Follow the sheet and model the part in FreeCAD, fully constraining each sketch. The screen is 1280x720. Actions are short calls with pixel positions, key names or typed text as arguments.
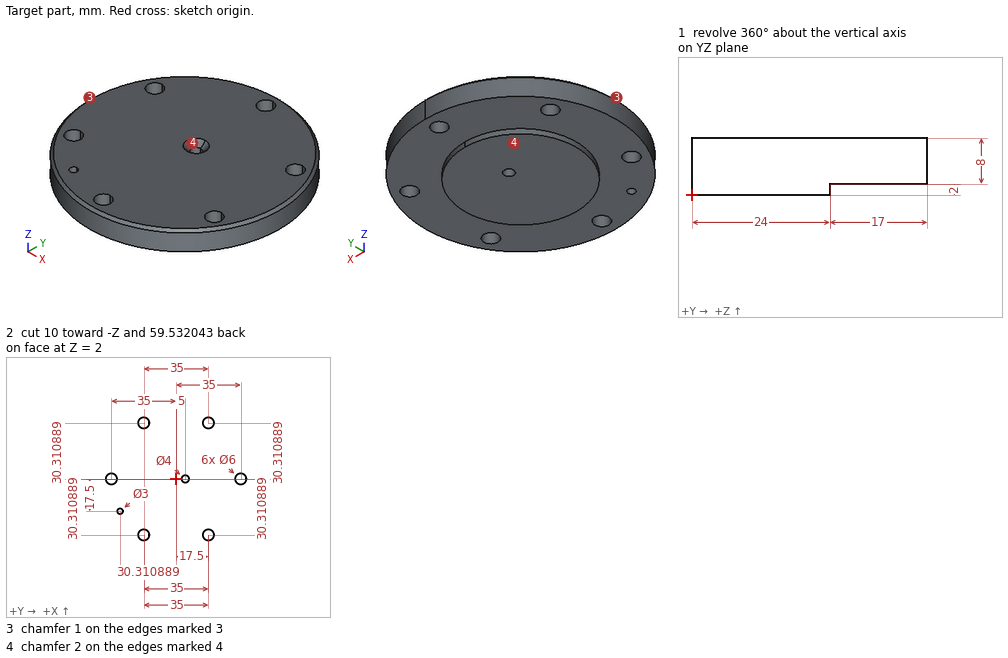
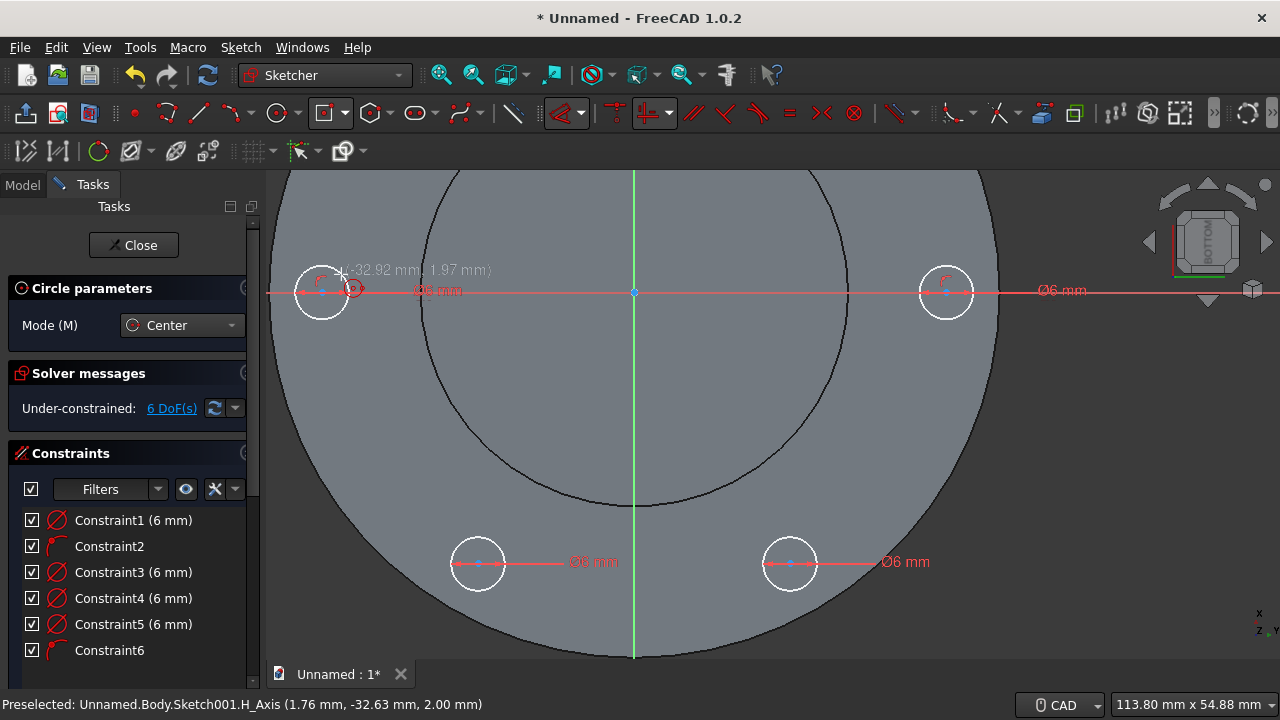
scroll(790, 563, down, 3)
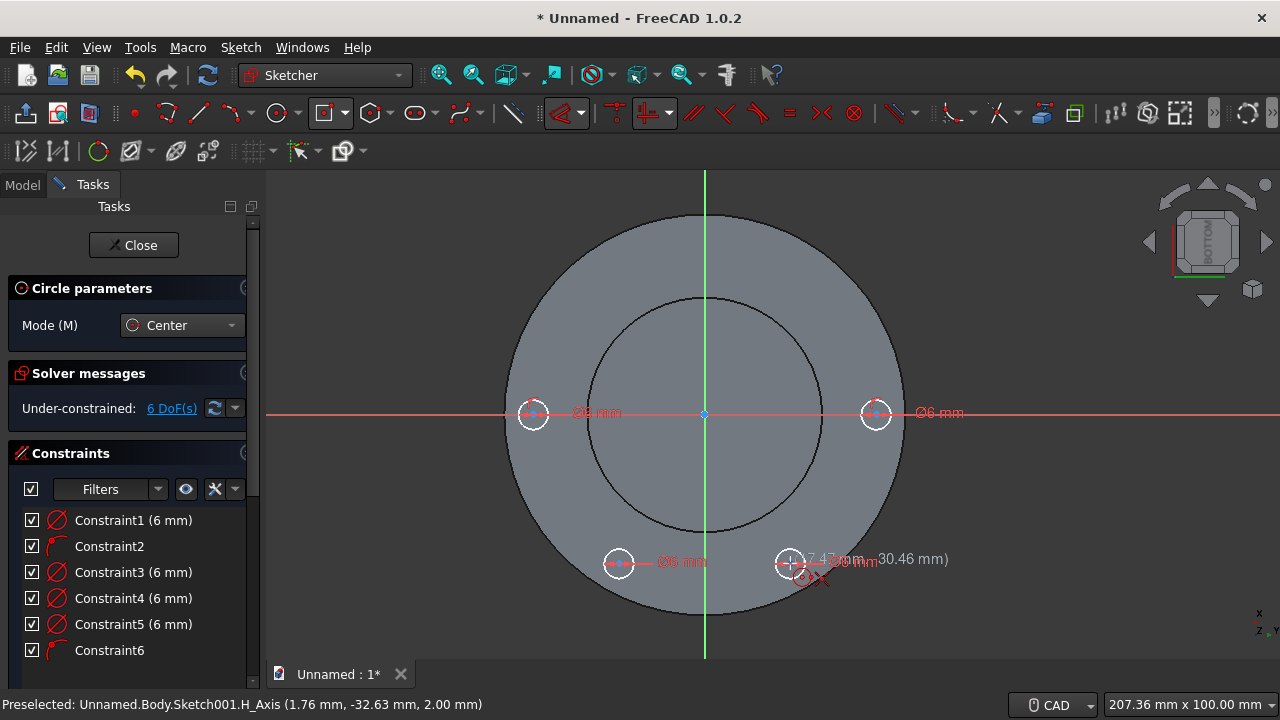
scroll(619, 267, up, 3)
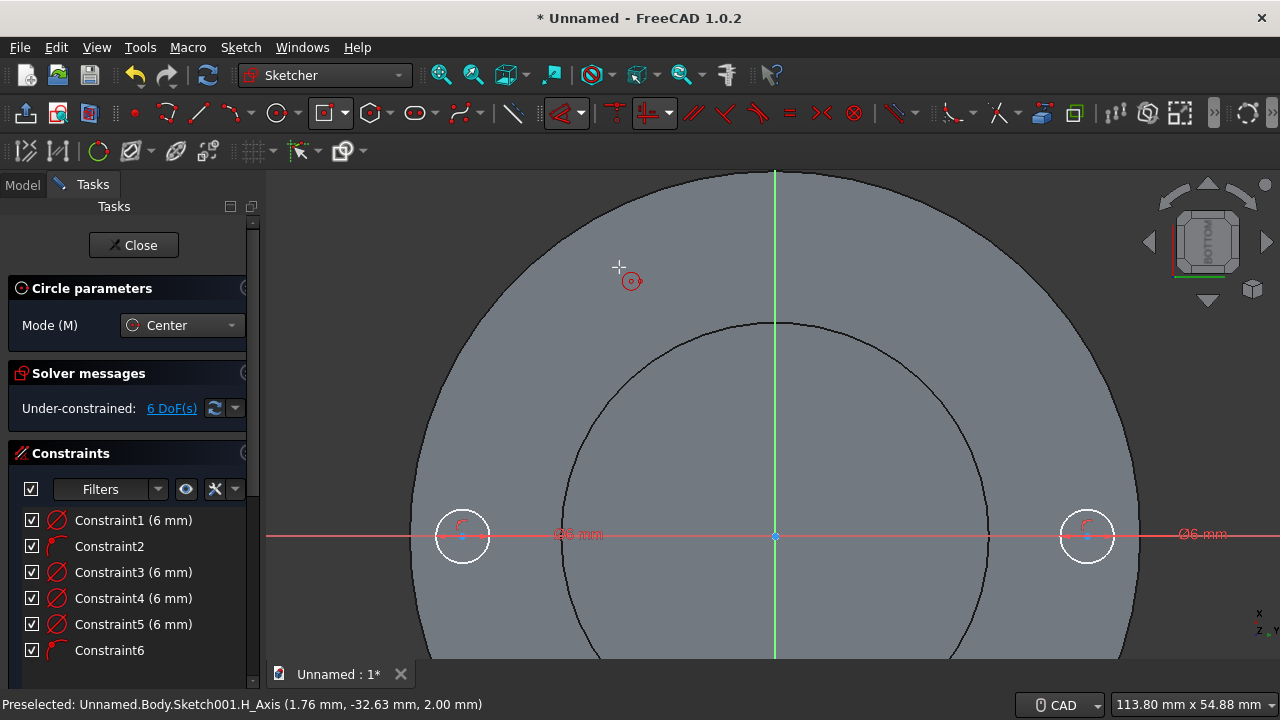
click(619, 266)
move(638, 247)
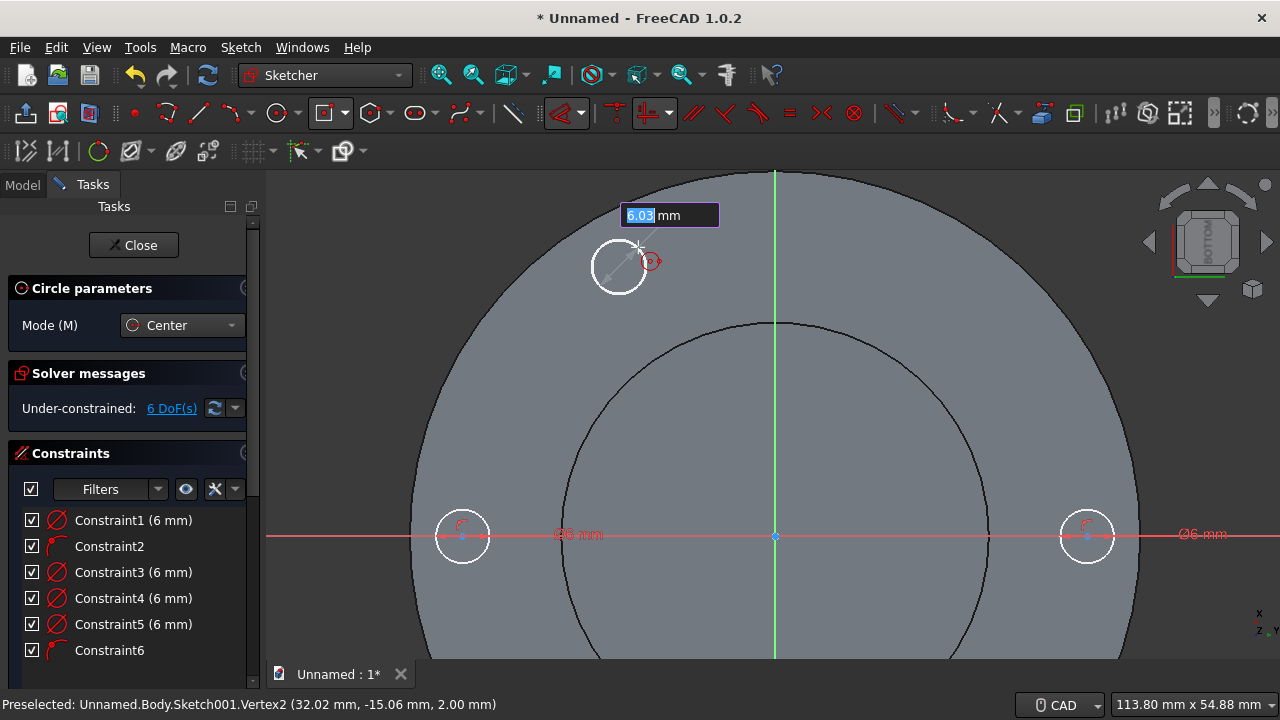
text(6)
key(Return)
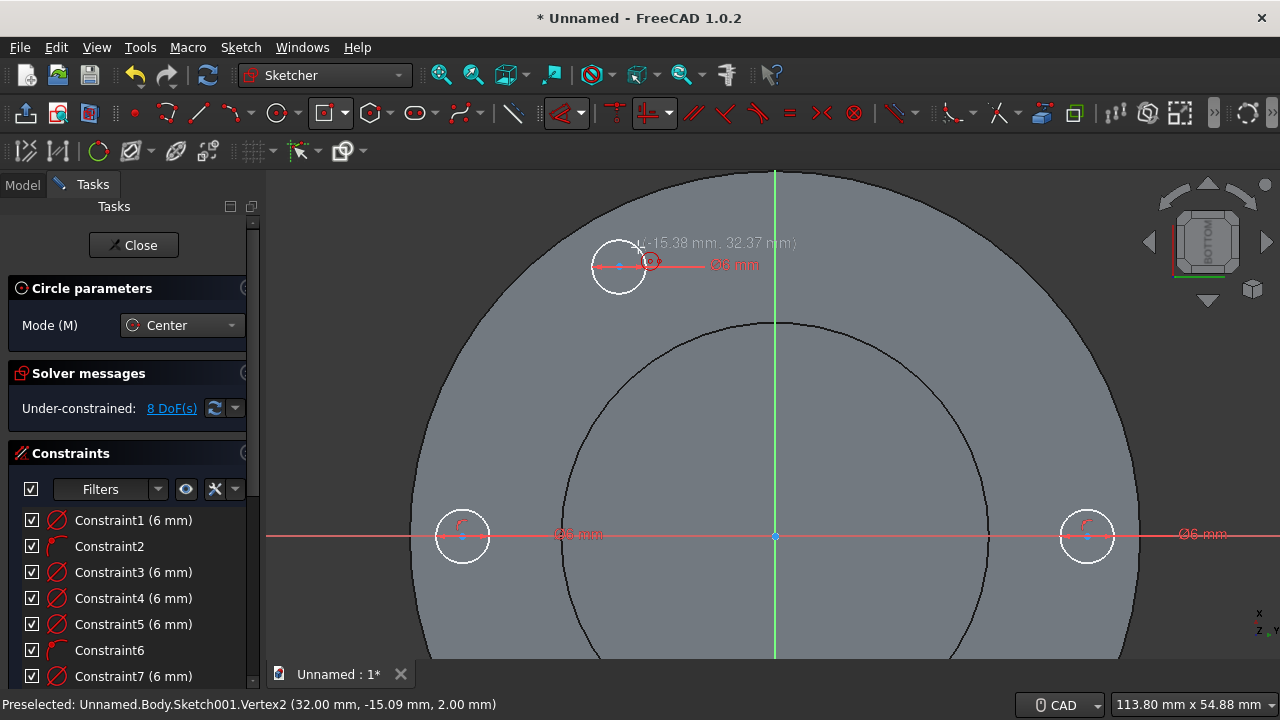
click(931, 266)
move(950, 247)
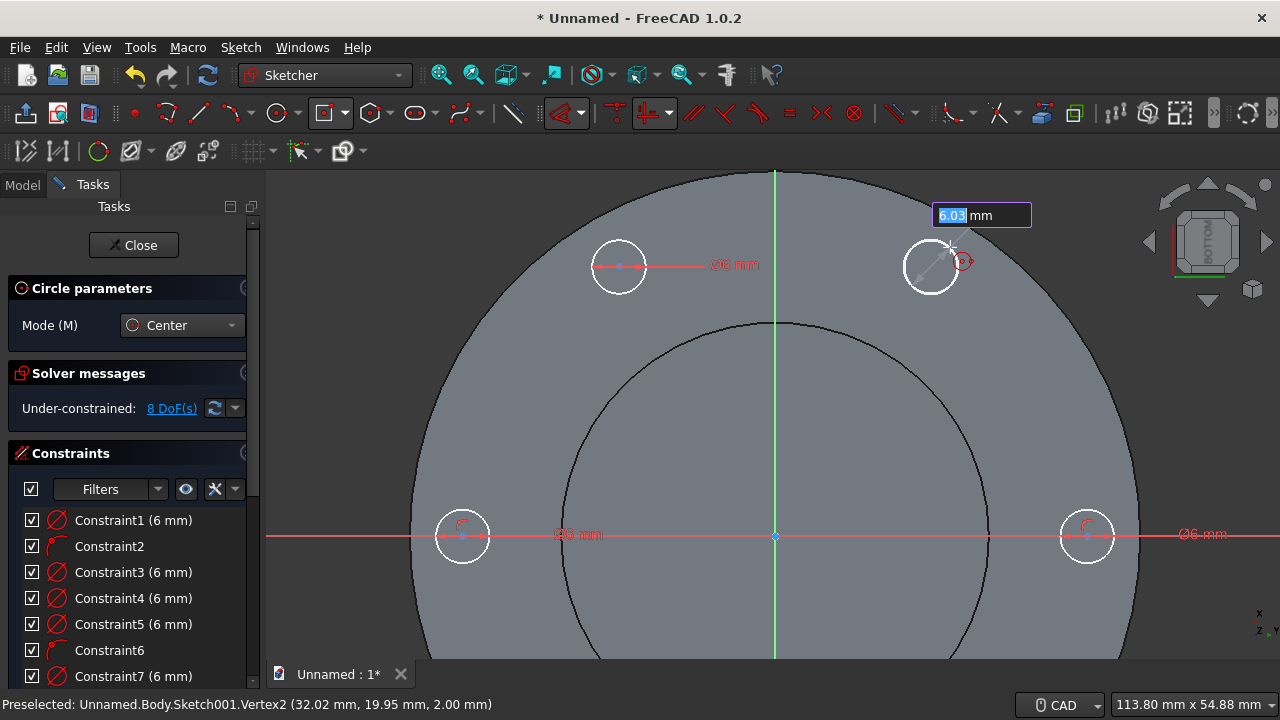
text(6)
key(Return)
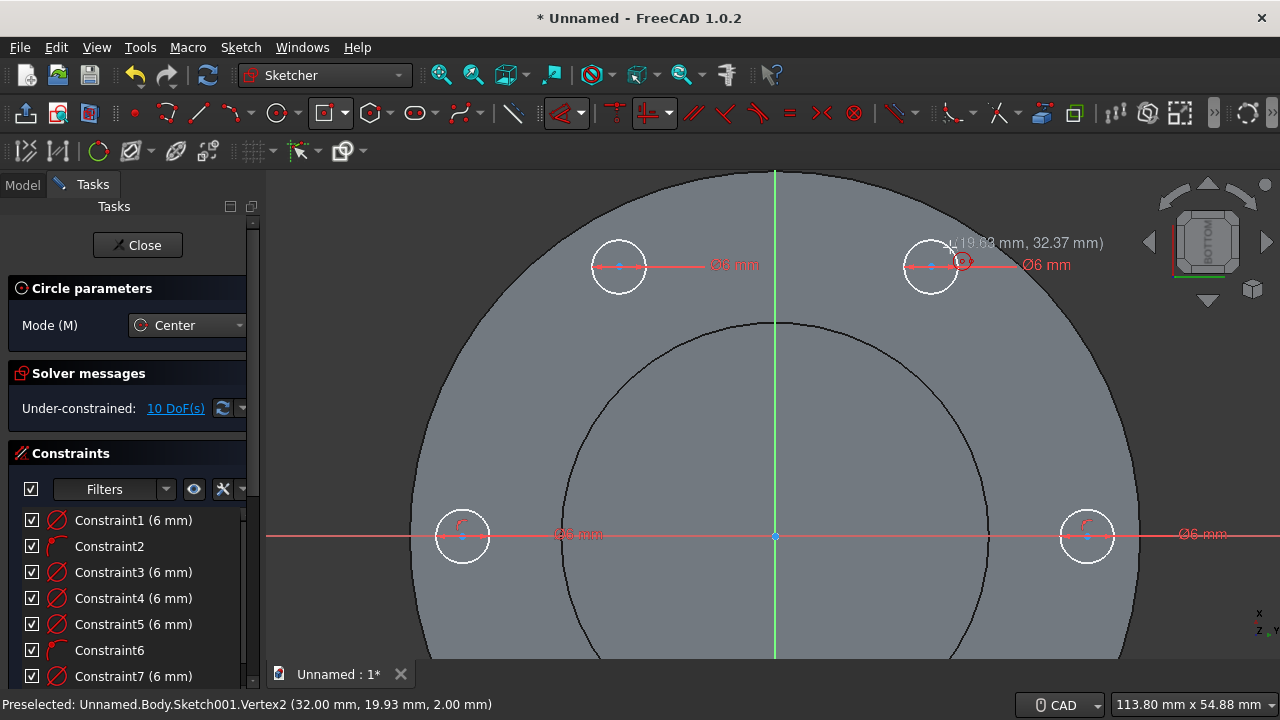
scroll(619, 266, down, 3)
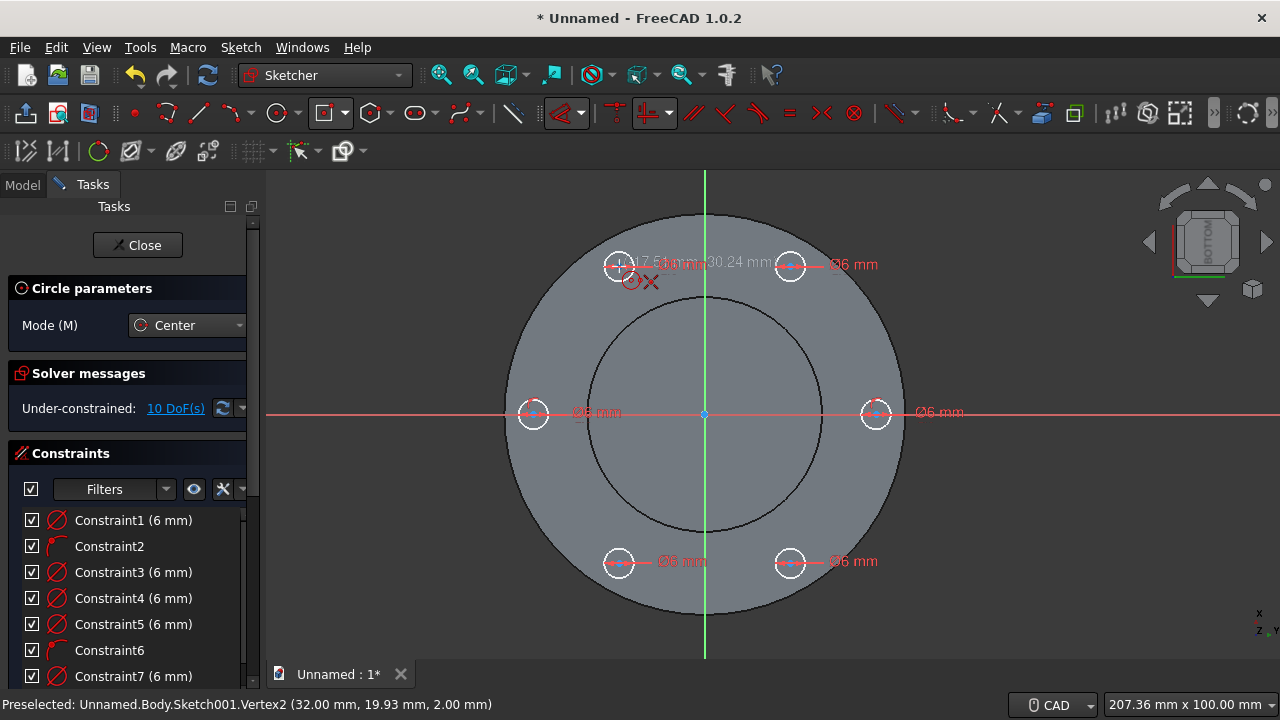
scroll(557, 500, up, 6)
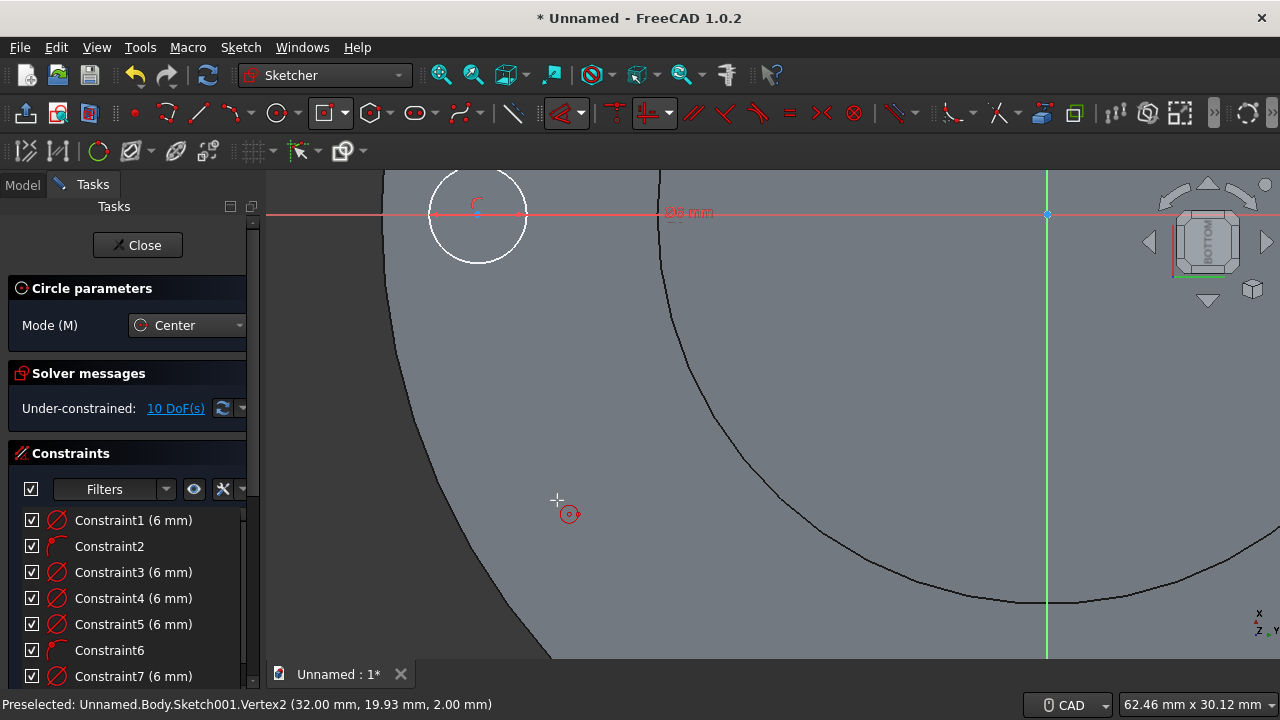
click(555, 499)
move(572, 481)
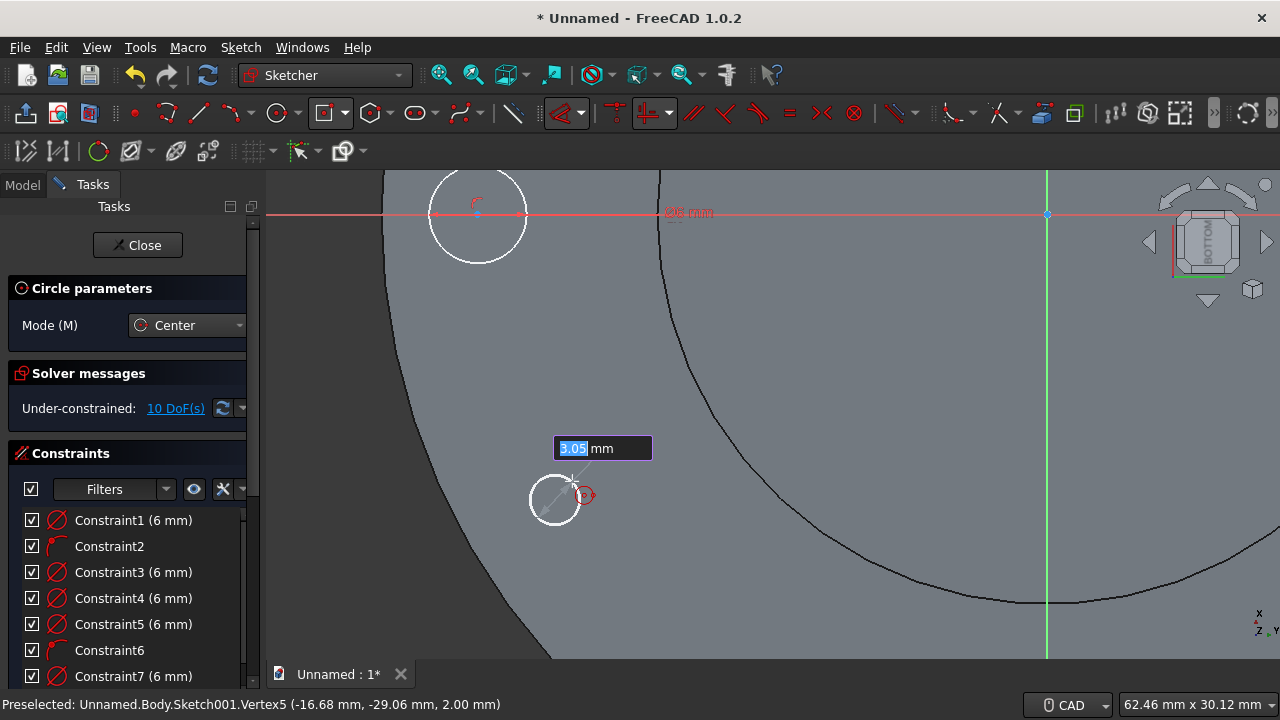
text(3)
key(Return)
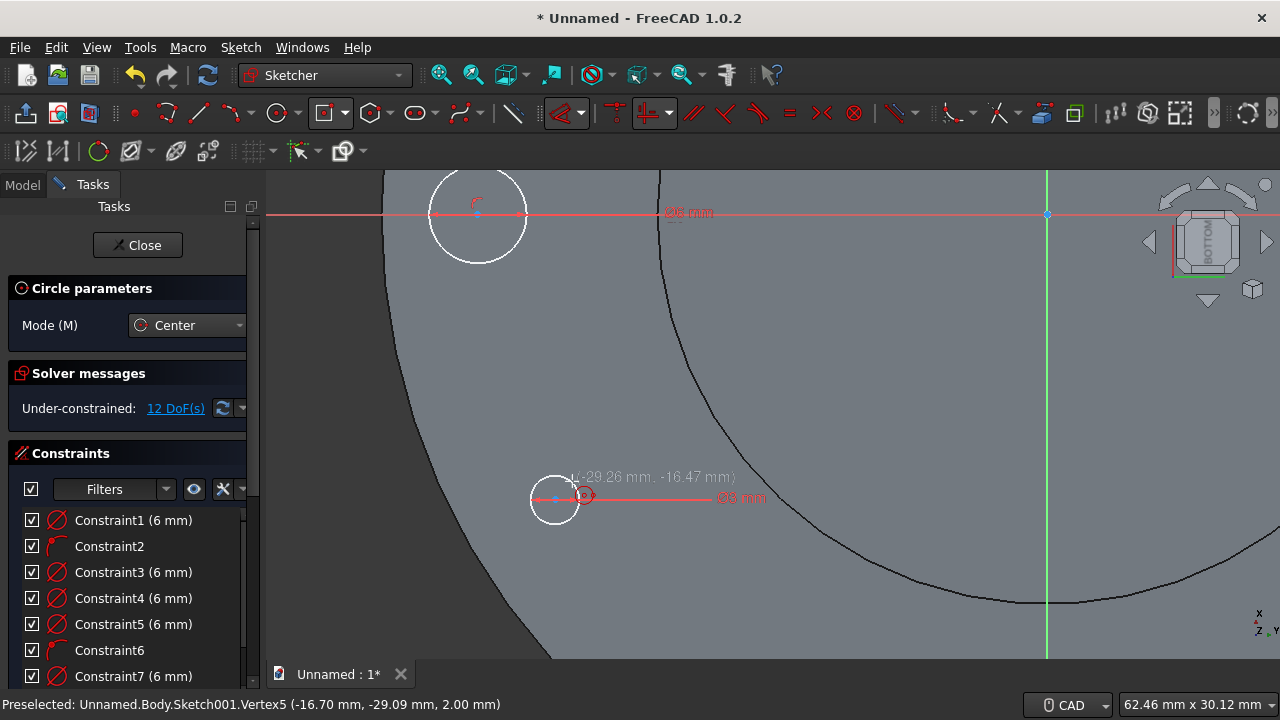
scroll(557, 501, down, 6)